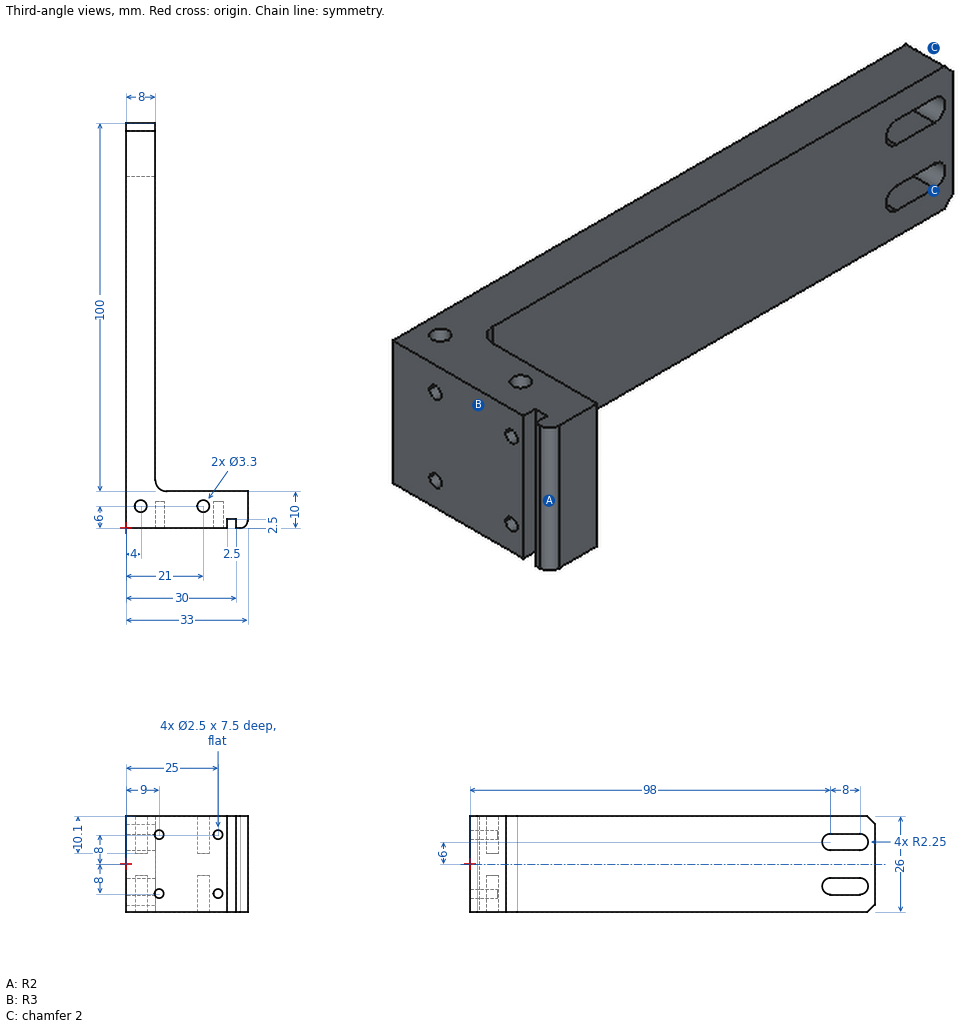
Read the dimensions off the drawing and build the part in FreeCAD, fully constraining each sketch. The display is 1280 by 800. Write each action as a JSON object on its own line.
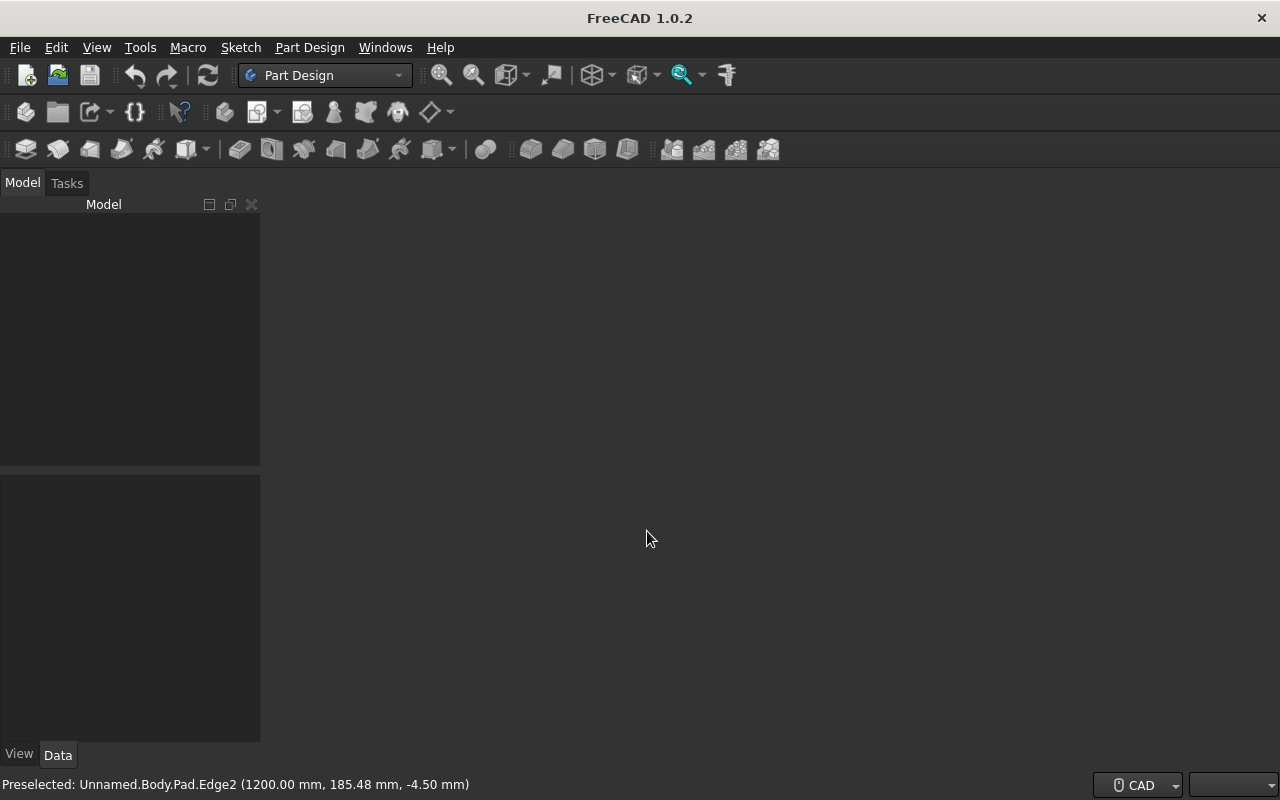
{"action": "left_click", "coordinate": [26, 76]}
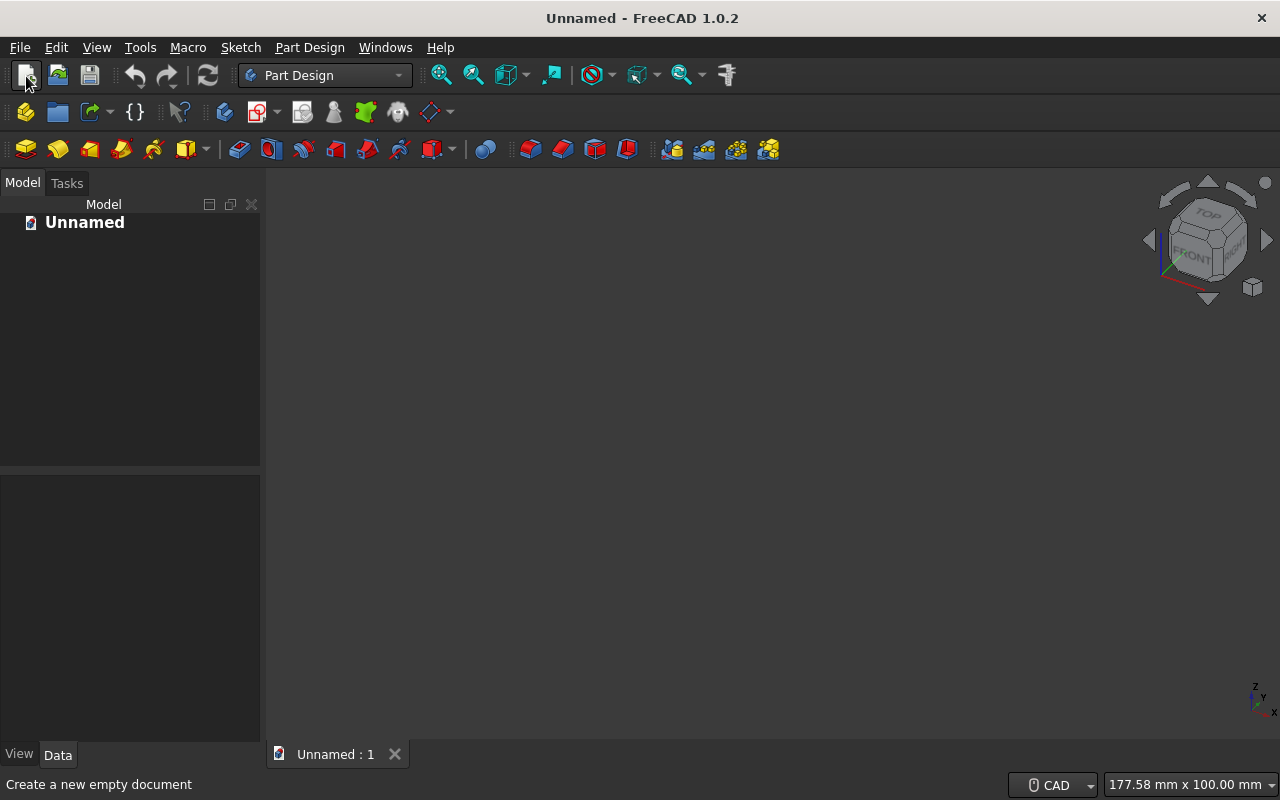
{"action": "left_click", "coordinate": [258, 112]}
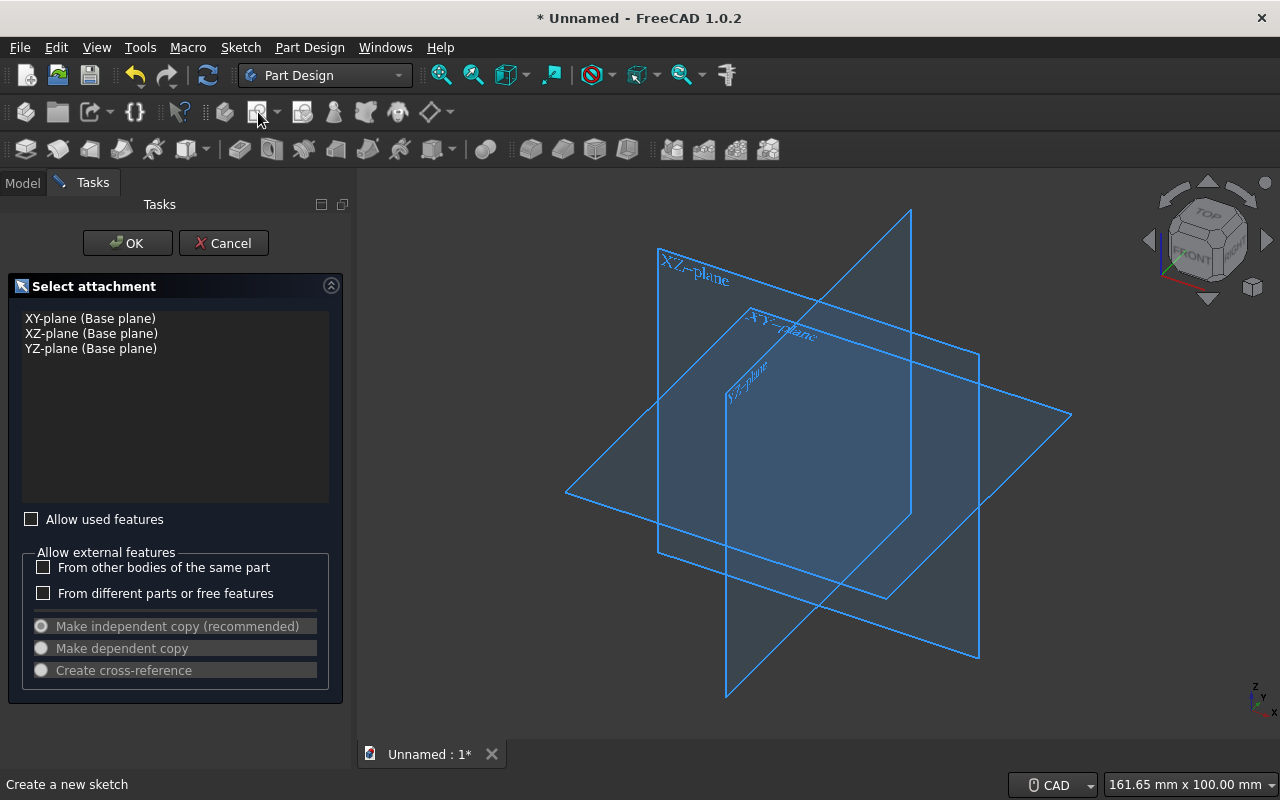
{"action": "left_click", "coordinate": [82, 318]}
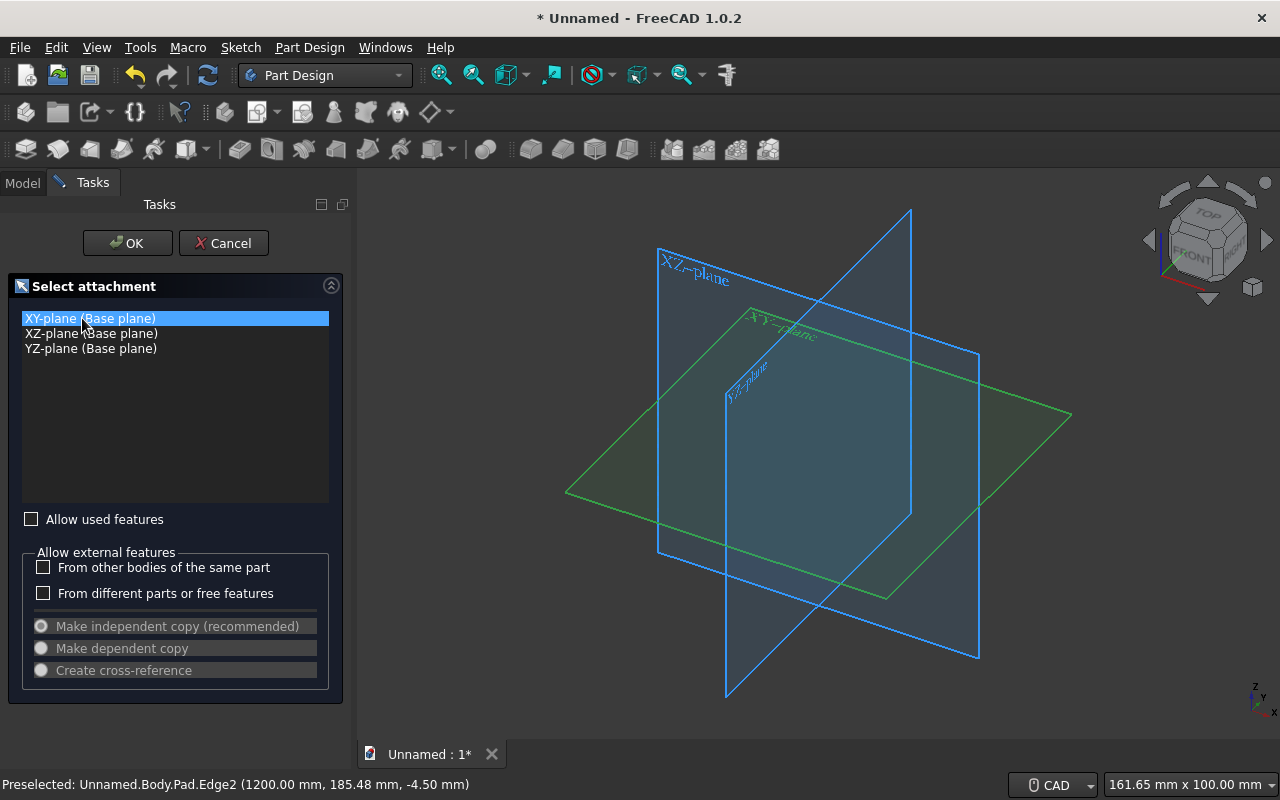
{"action": "left_click", "coordinate": [128, 243]}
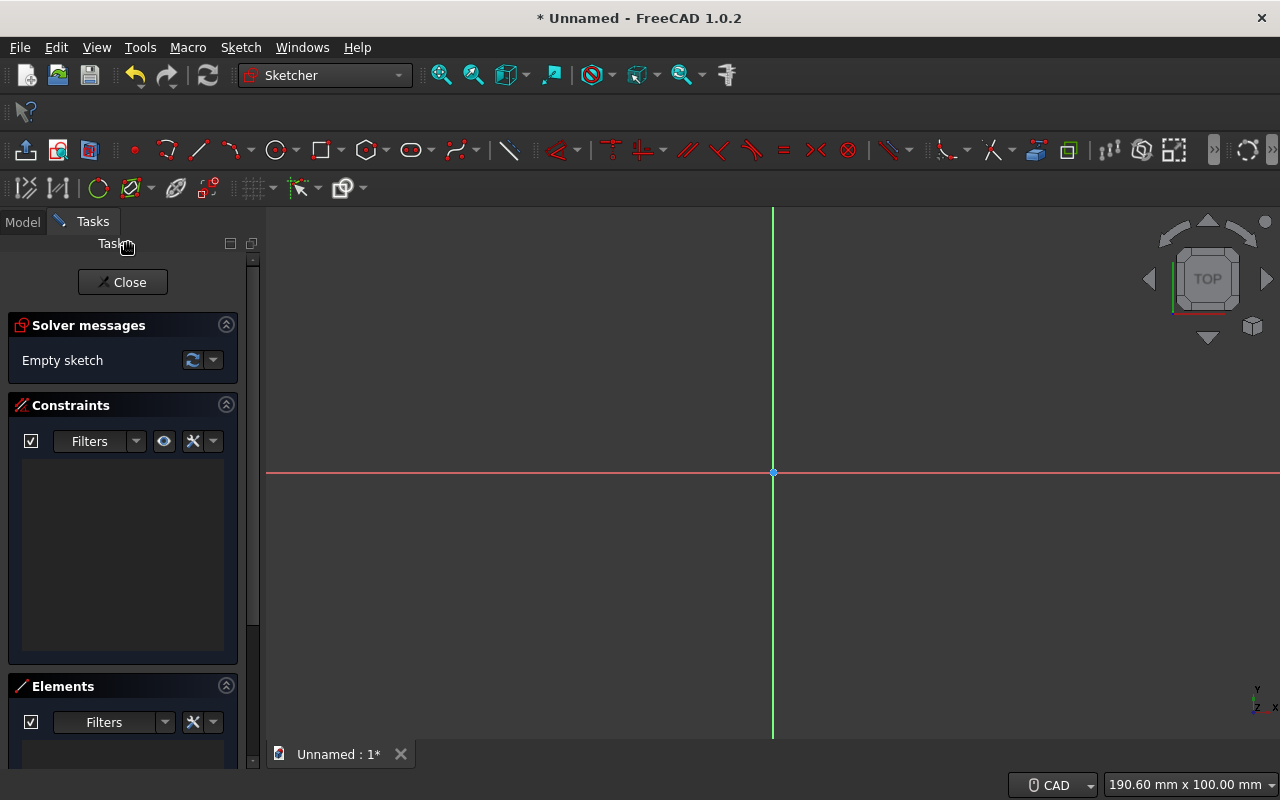
{"action": "scroll", "coordinate": [577, 711], "scroll_direction": "down", "scroll_amount": 4}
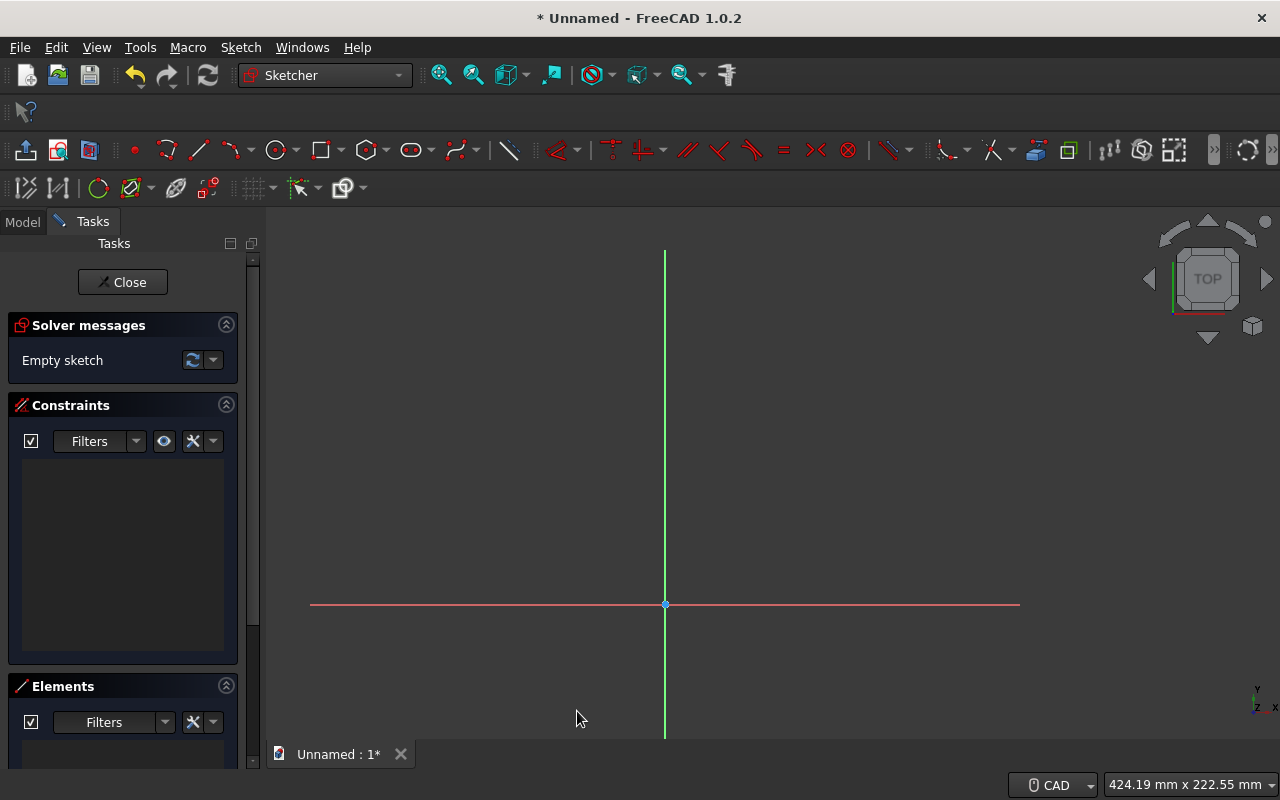
{"action": "left_click", "coordinate": [168, 150]}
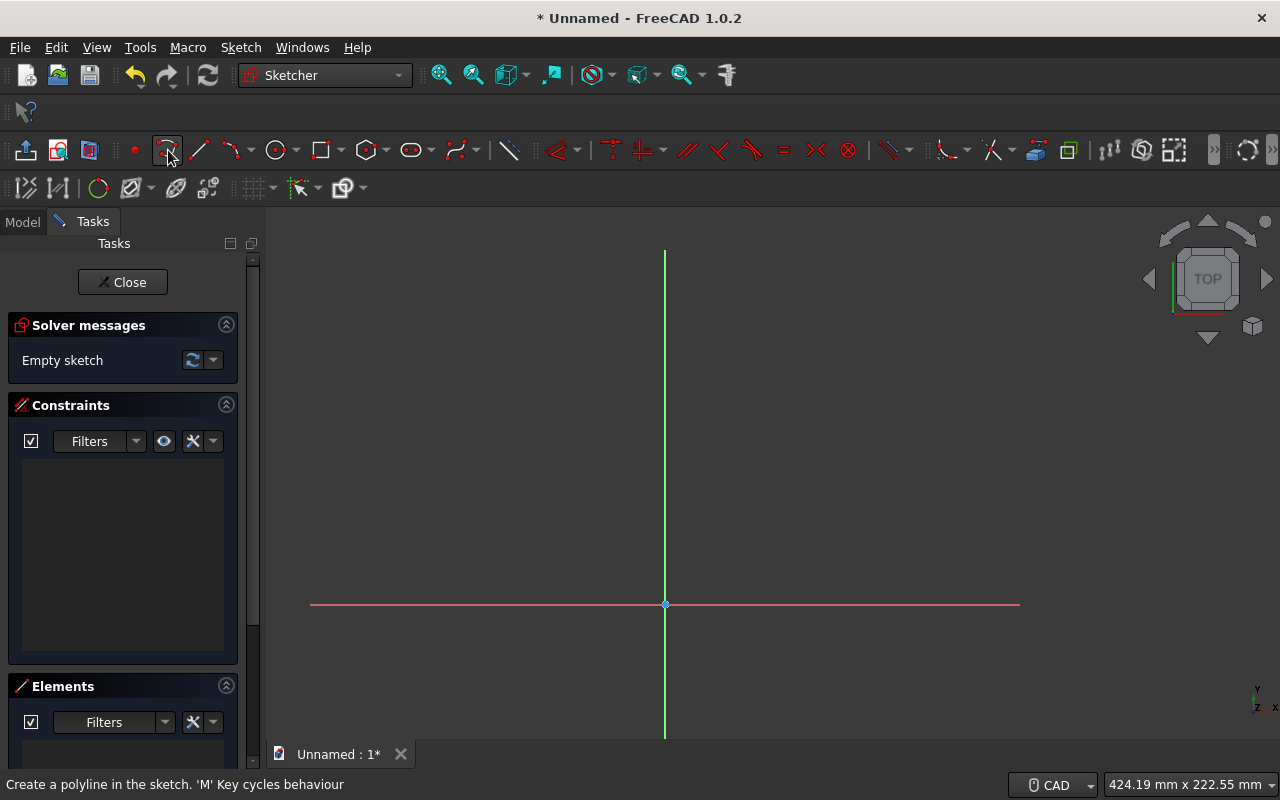
{"action": "left_click", "coordinate": [665, 605]}
{"action": "left_click", "coordinate": [744, 596]}
{"action": "left_click", "coordinate": [744, 581]}
{"action": "left_click", "coordinate": [684, 581]}
{"action": "left_click", "coordinate": [684, 342]}
{"action": "left_click", "coordinate": [674, 342]}
{"action": "left_click", "coordinate": [665, 605]}
{"action": "key", "text": "Escape"}
{"action": "key", "text": "Escape"}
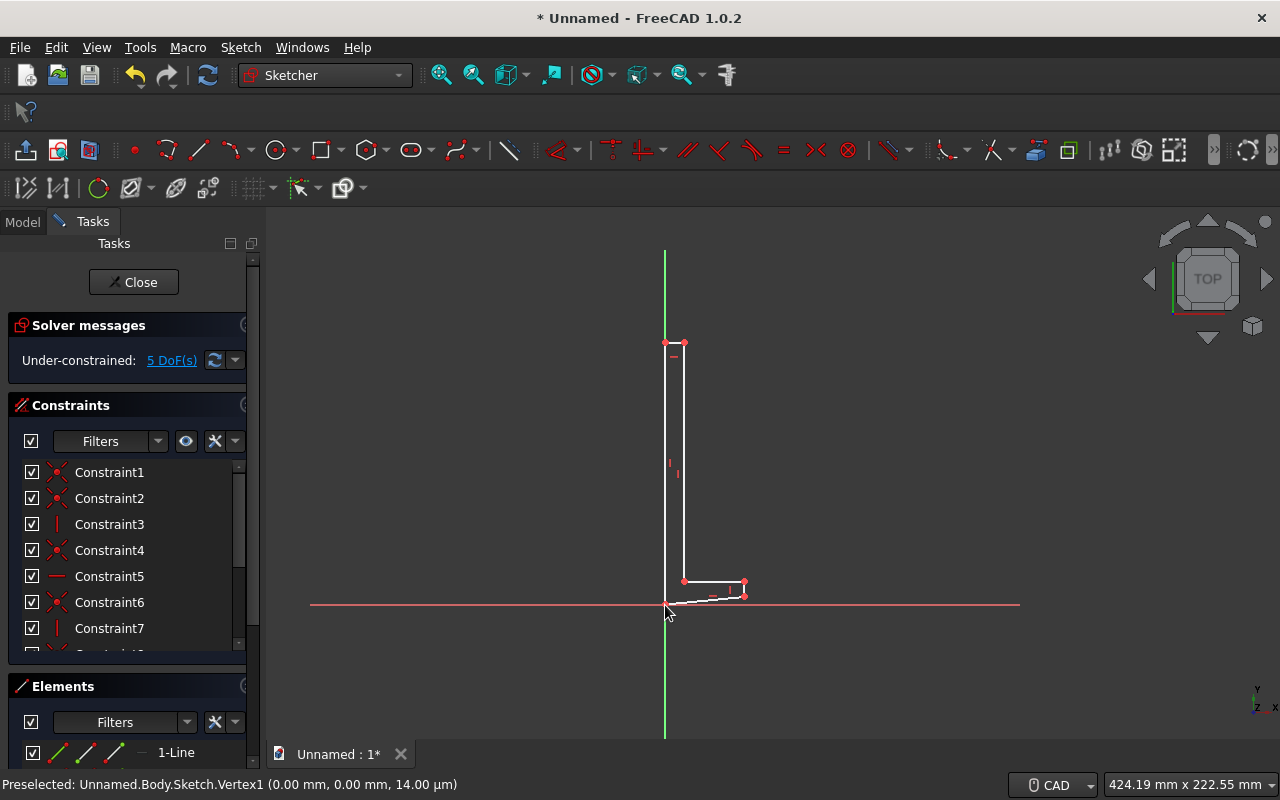
{"action": "left_click", "coordinate": [689, 602]}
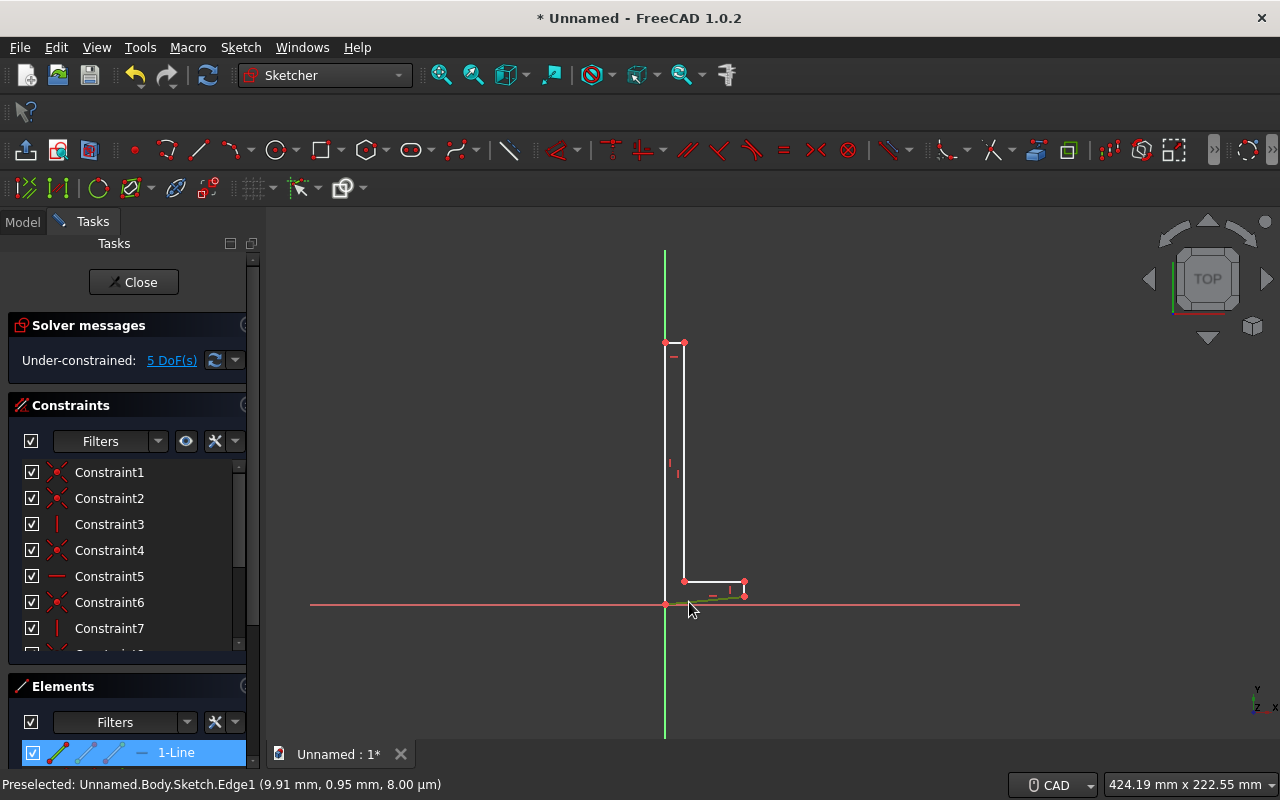
{"action": "left_click", "coordinate": [666, 150]}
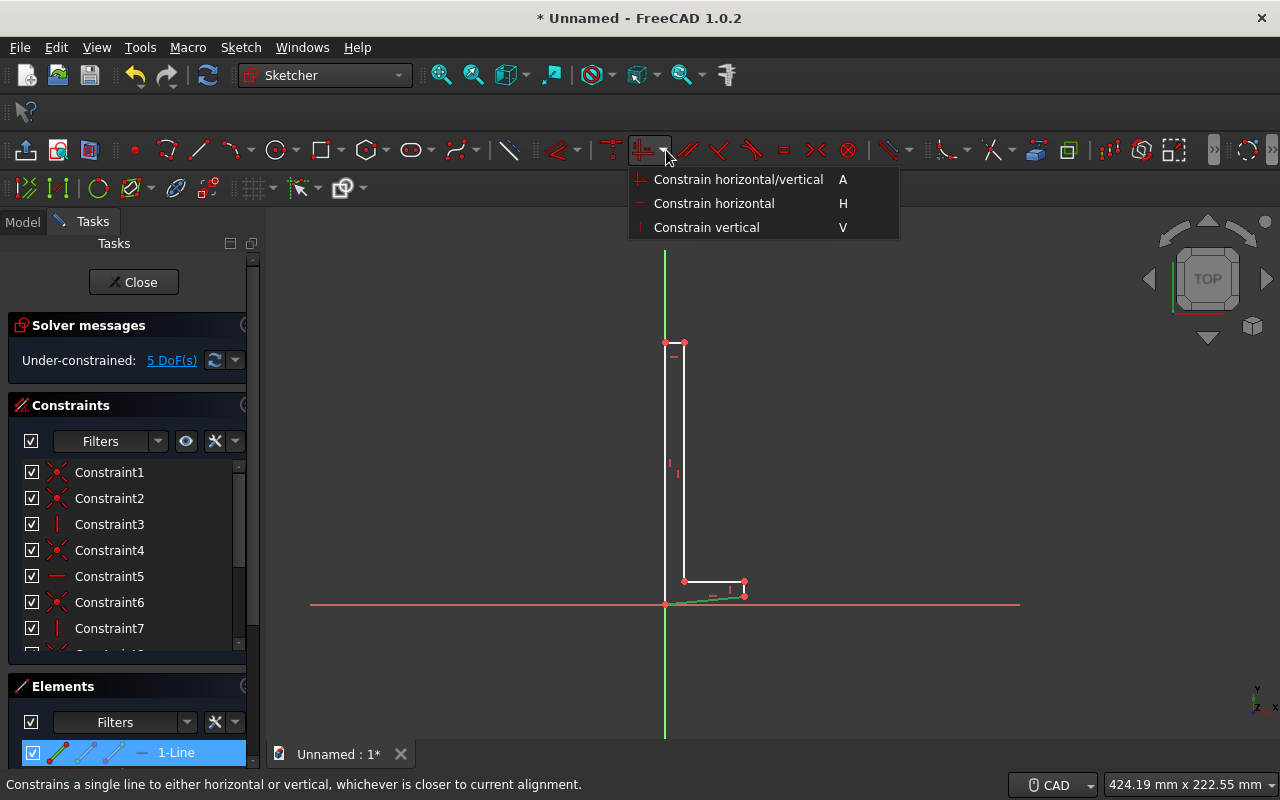
{"action": "left_click", "coordinate": [764, 203]}